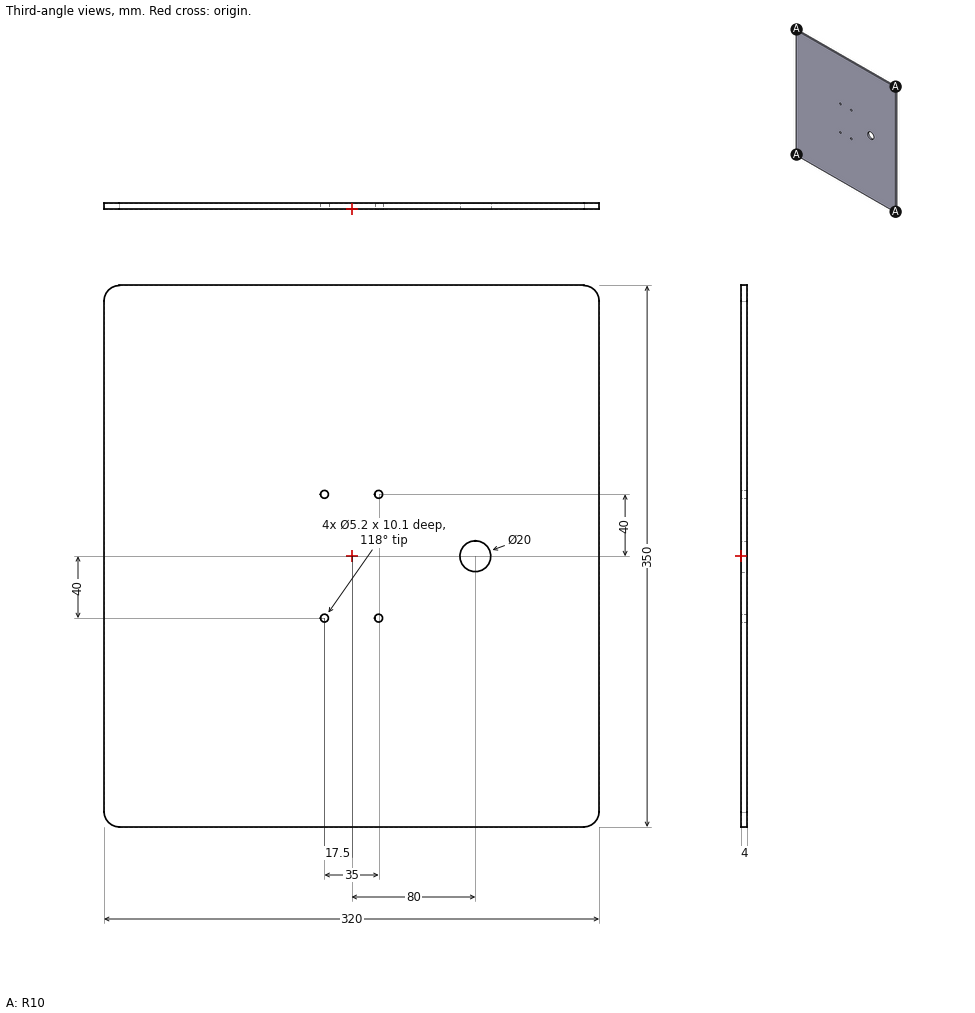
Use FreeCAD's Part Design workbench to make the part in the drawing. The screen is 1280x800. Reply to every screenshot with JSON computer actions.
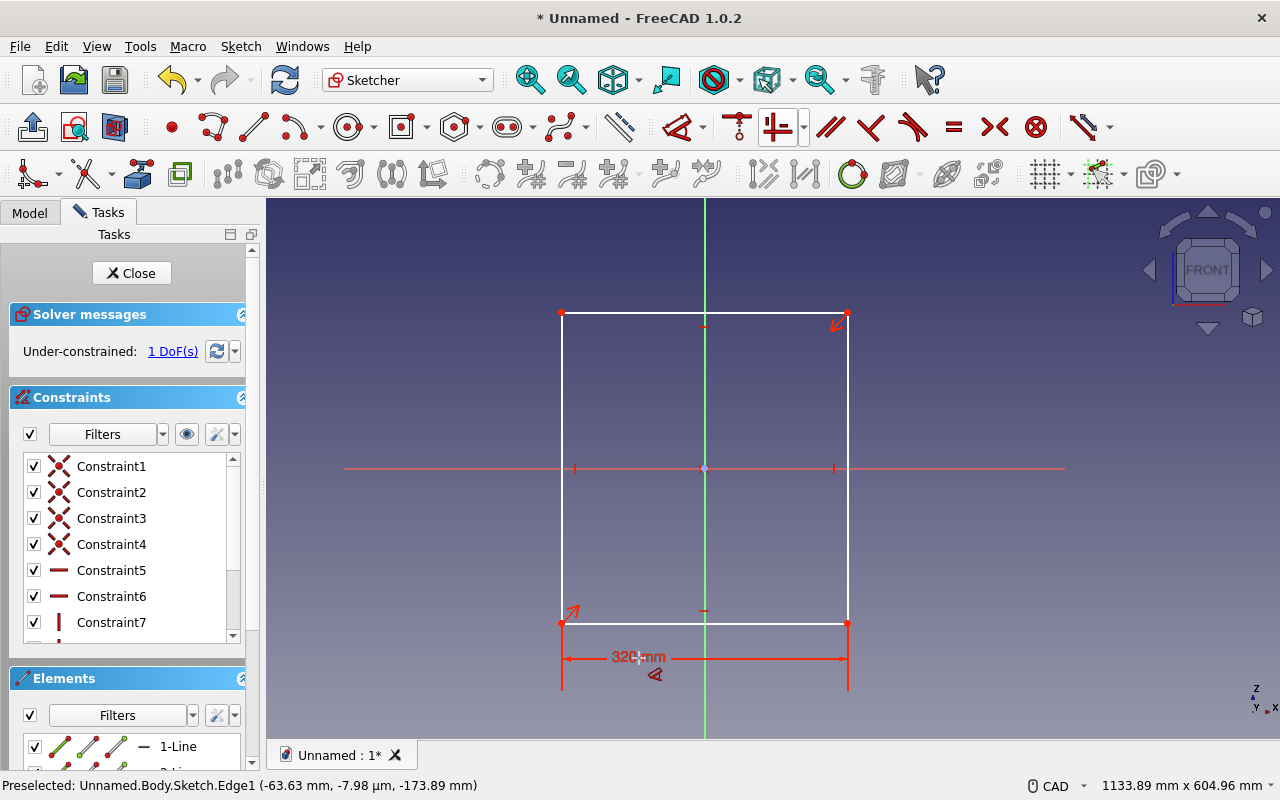
{"action": "left_click", "coordinate": [848, 531]}
{"action": "left_click", "coordinate": [882, 397]}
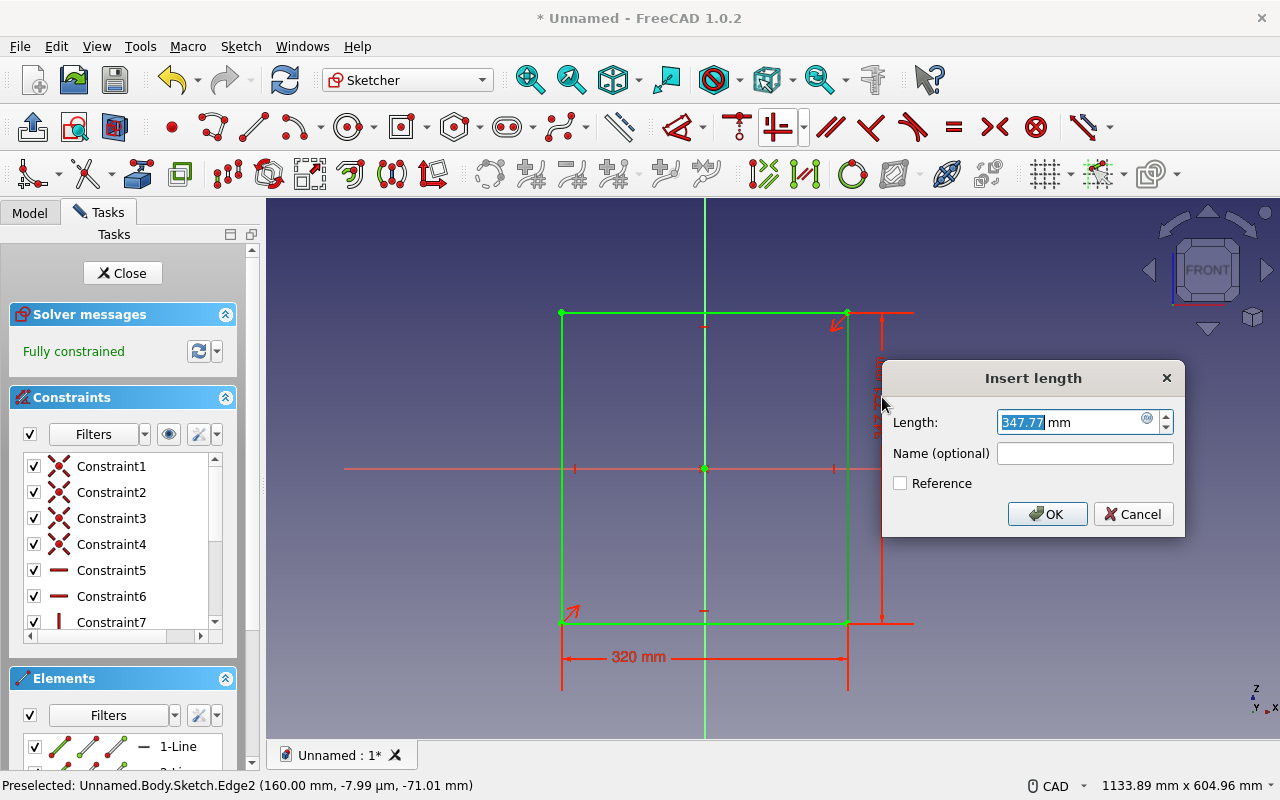
{"action": "type", "text": "350"}
{"action": "key", "text": "Return"}
{"action": "key", "text": "Escape"}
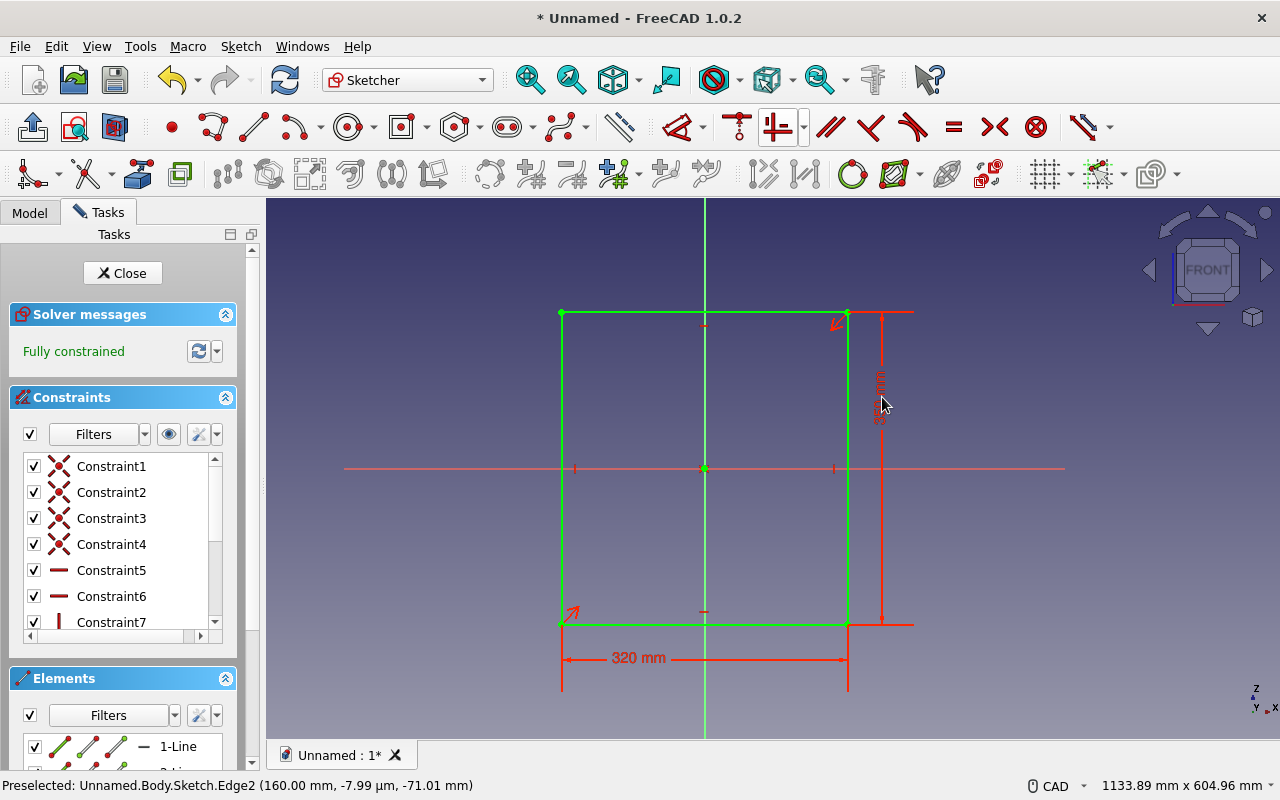
{"action": "left_click", "coordinate": [123, 273]}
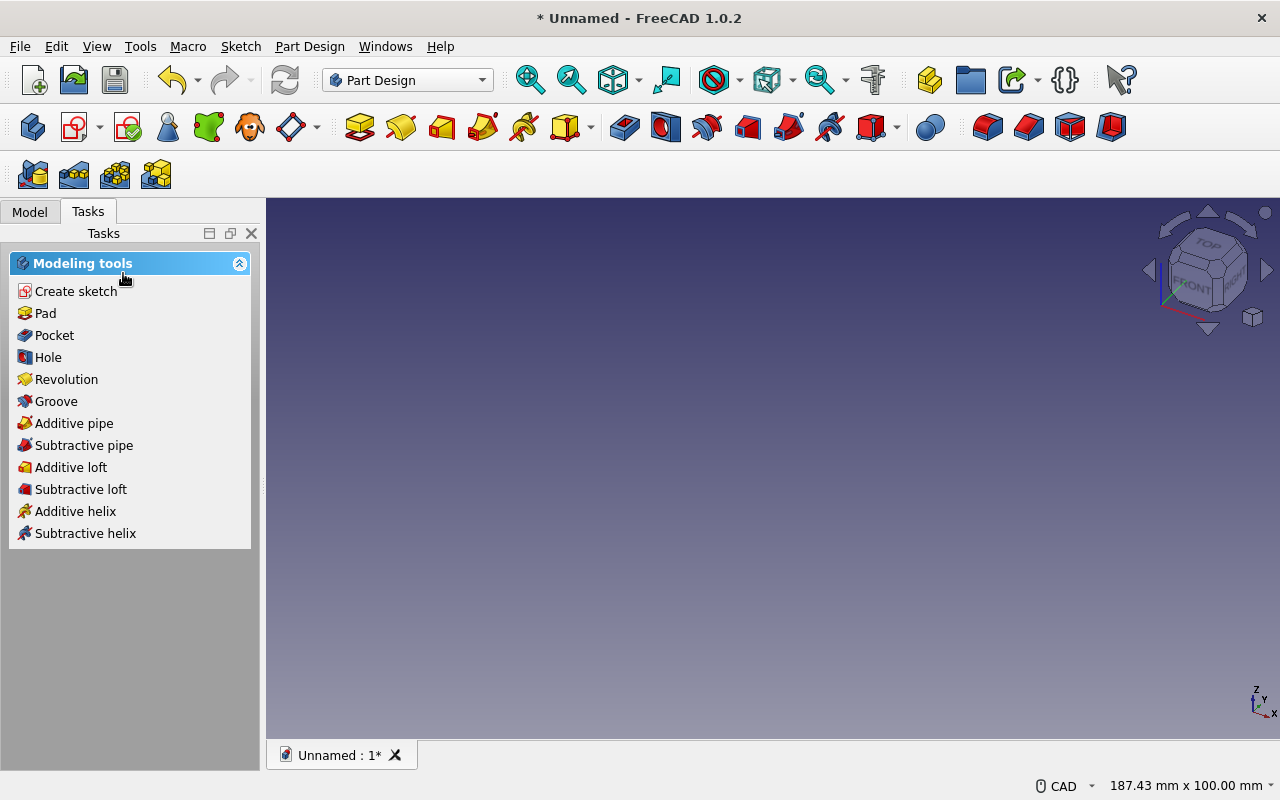
{"action": "left_click", "coordinate": [360, 128]}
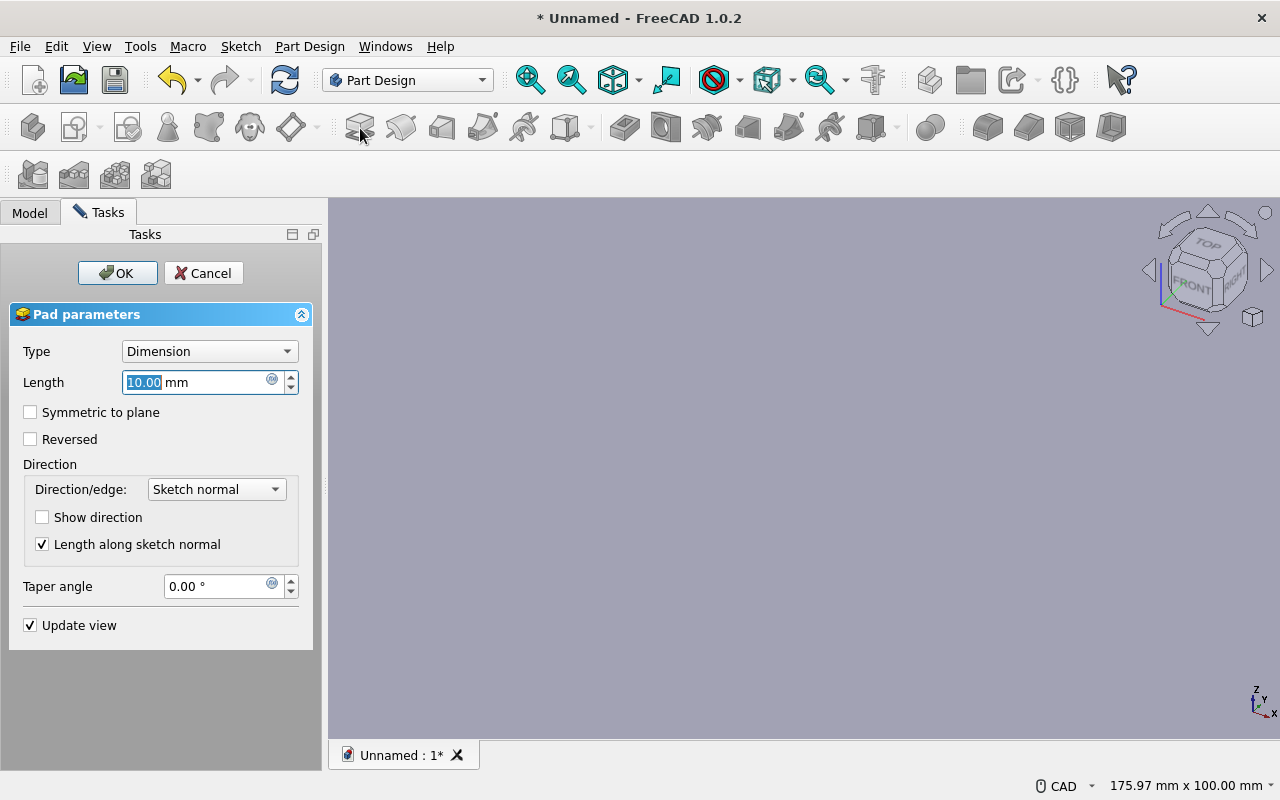
{"action": "type", "text": "4"}
{"action": "key", "text": "Tab"}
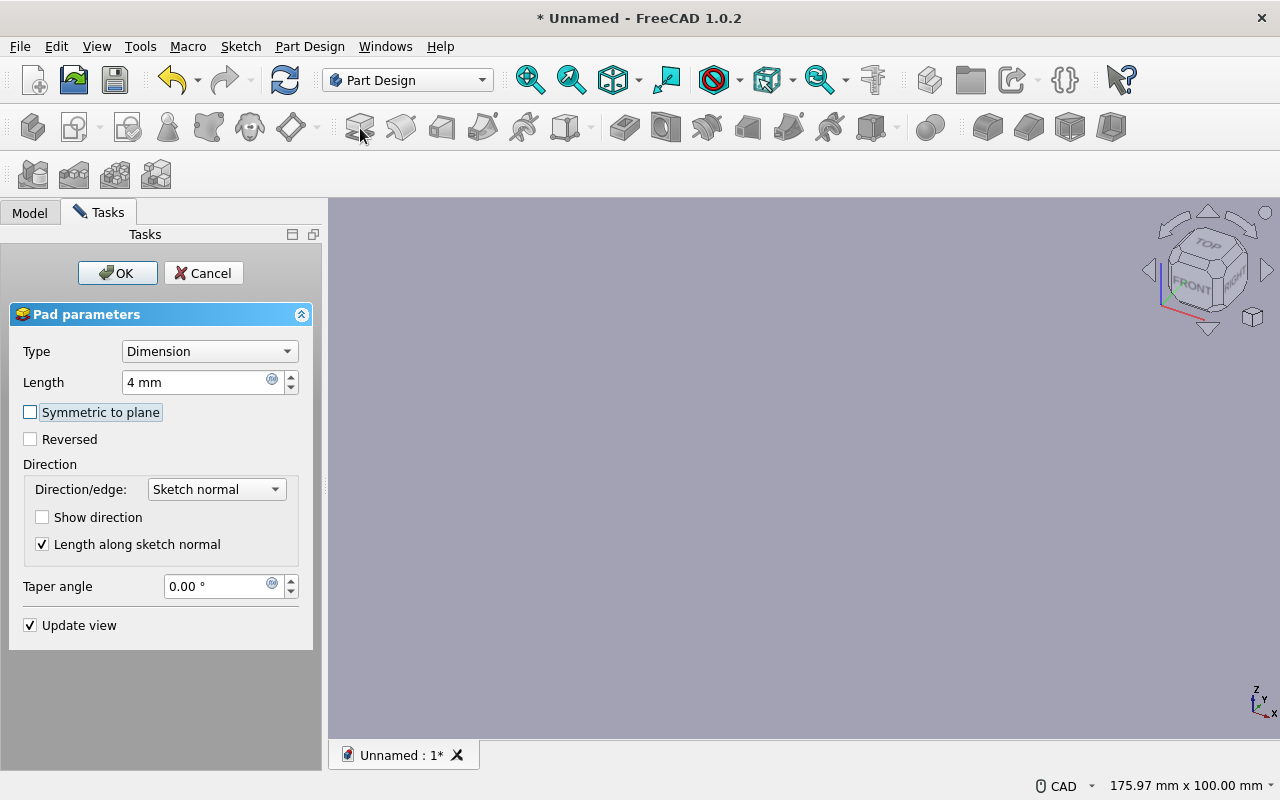
{"action": "left_click", "coordinate": [31, 439]}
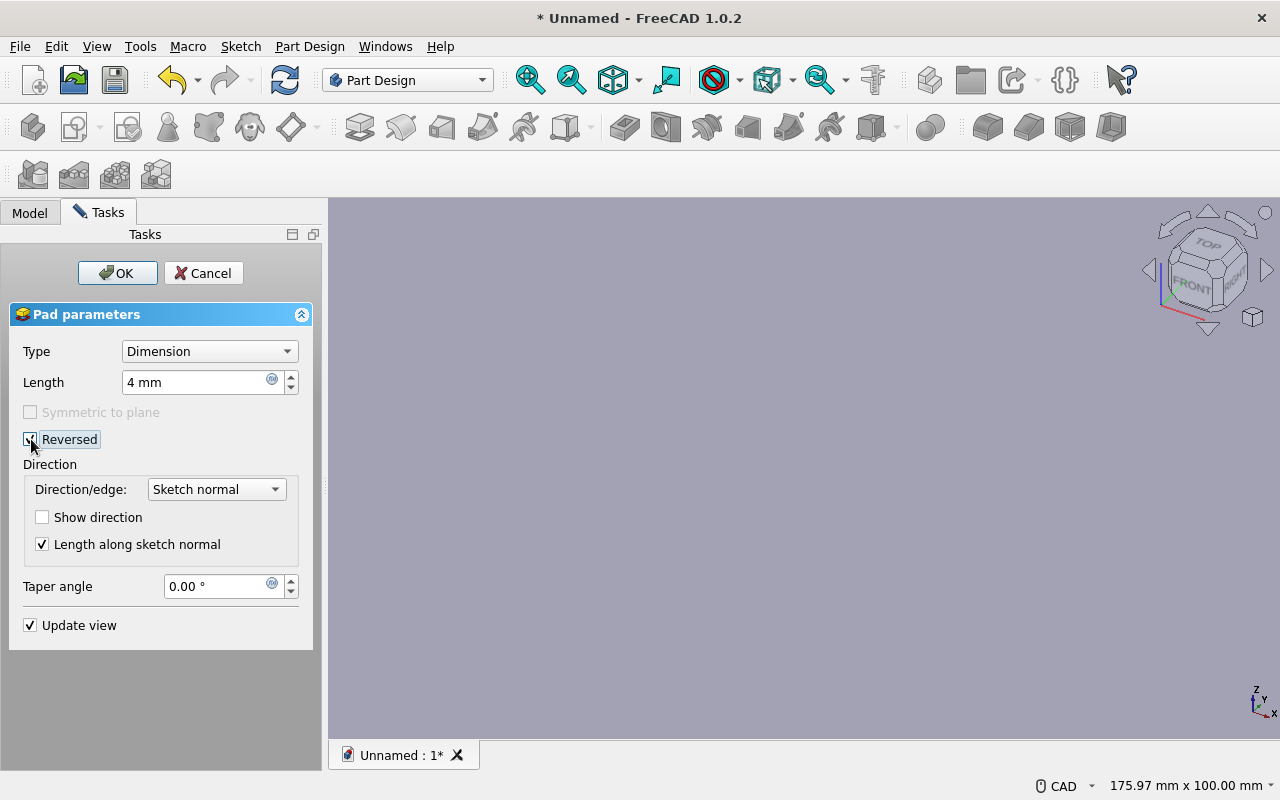
{"action": "left_click", "coordinate": [118, 273]}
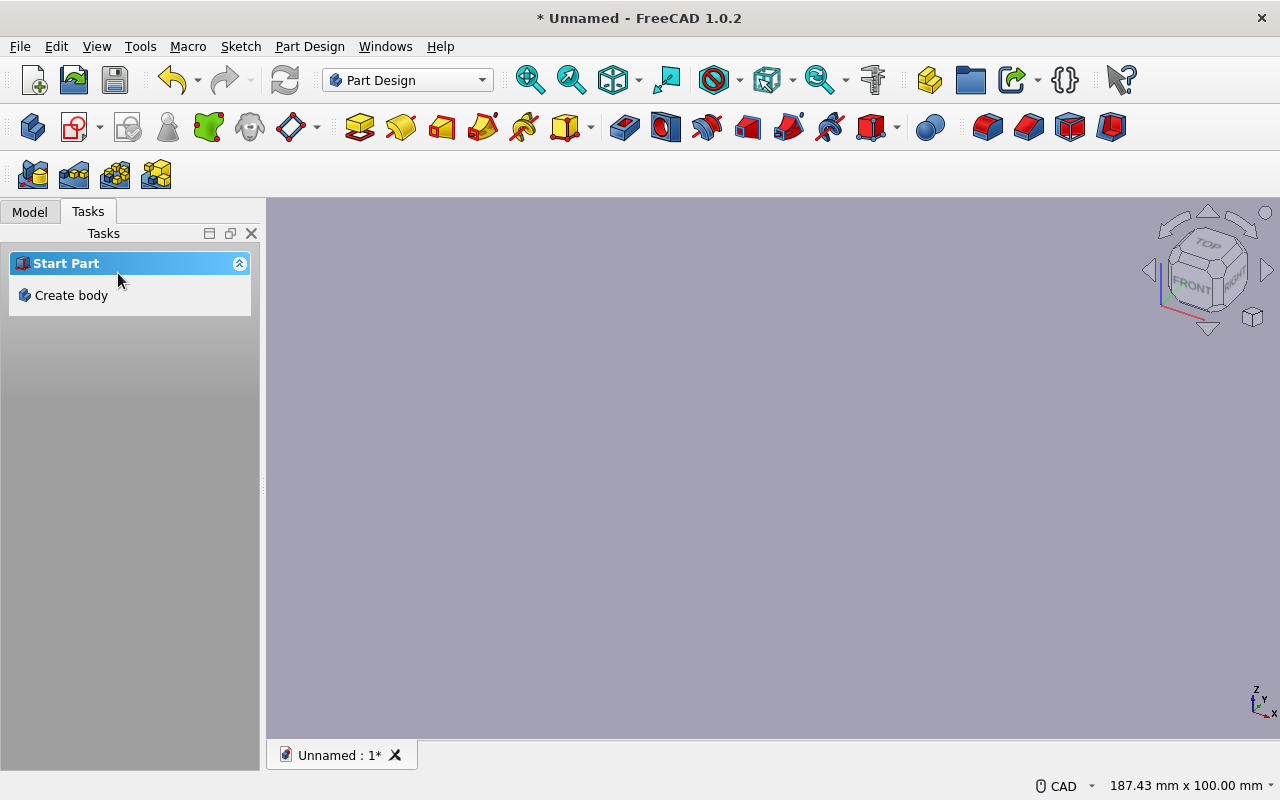
{"action": "left_click", "coordinate": [531, 80]}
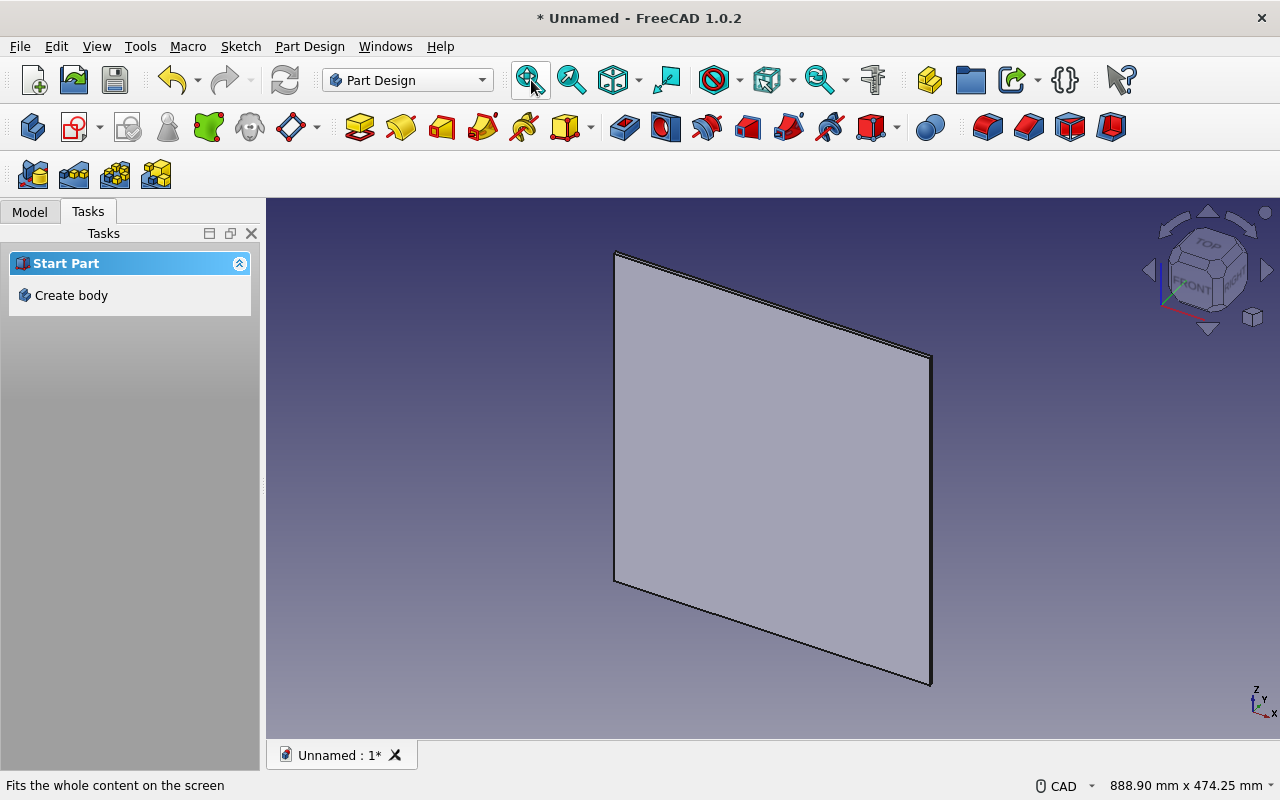
{"action": "key", "text": "4"}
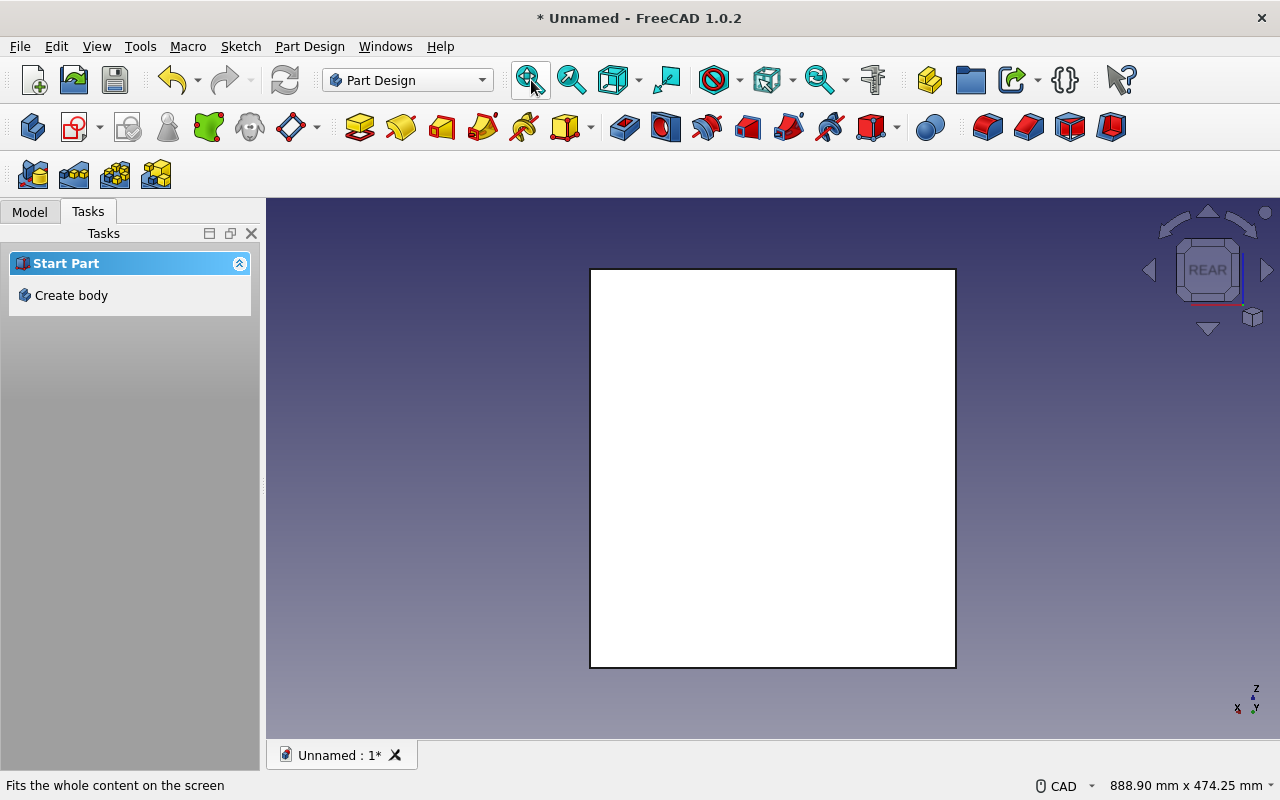
{"action": "left_click", "coordinate": [773, 468]}